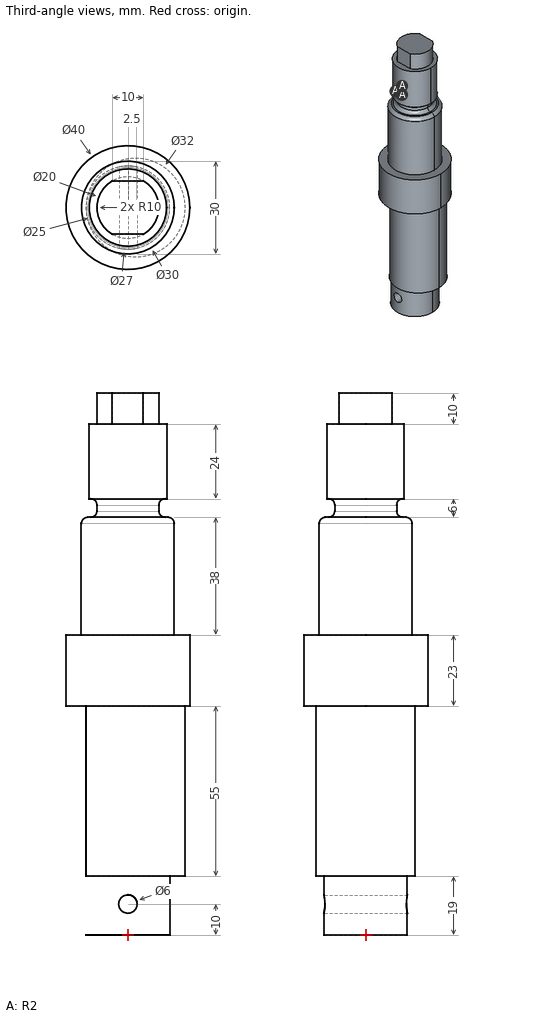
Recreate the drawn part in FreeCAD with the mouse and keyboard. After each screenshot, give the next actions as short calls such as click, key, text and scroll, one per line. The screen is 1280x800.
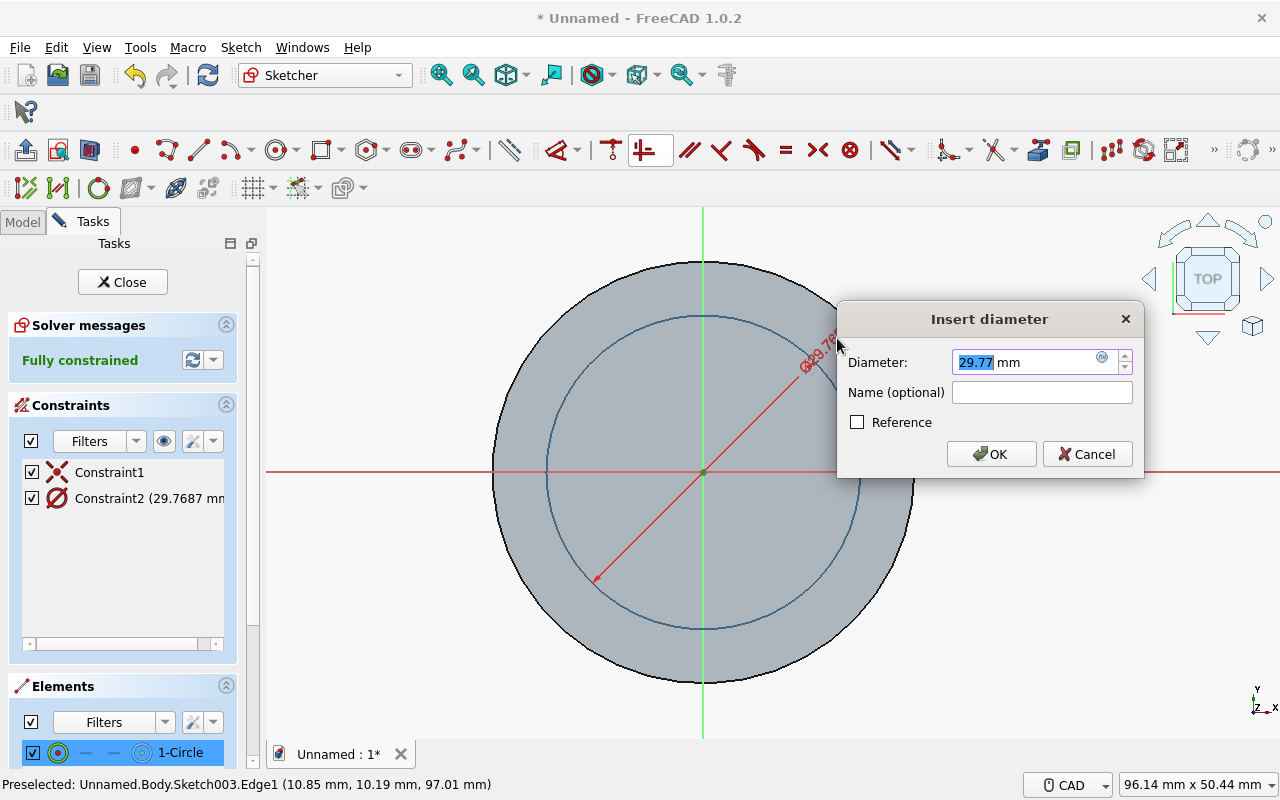
text(30)
key(Return)
key(Escape)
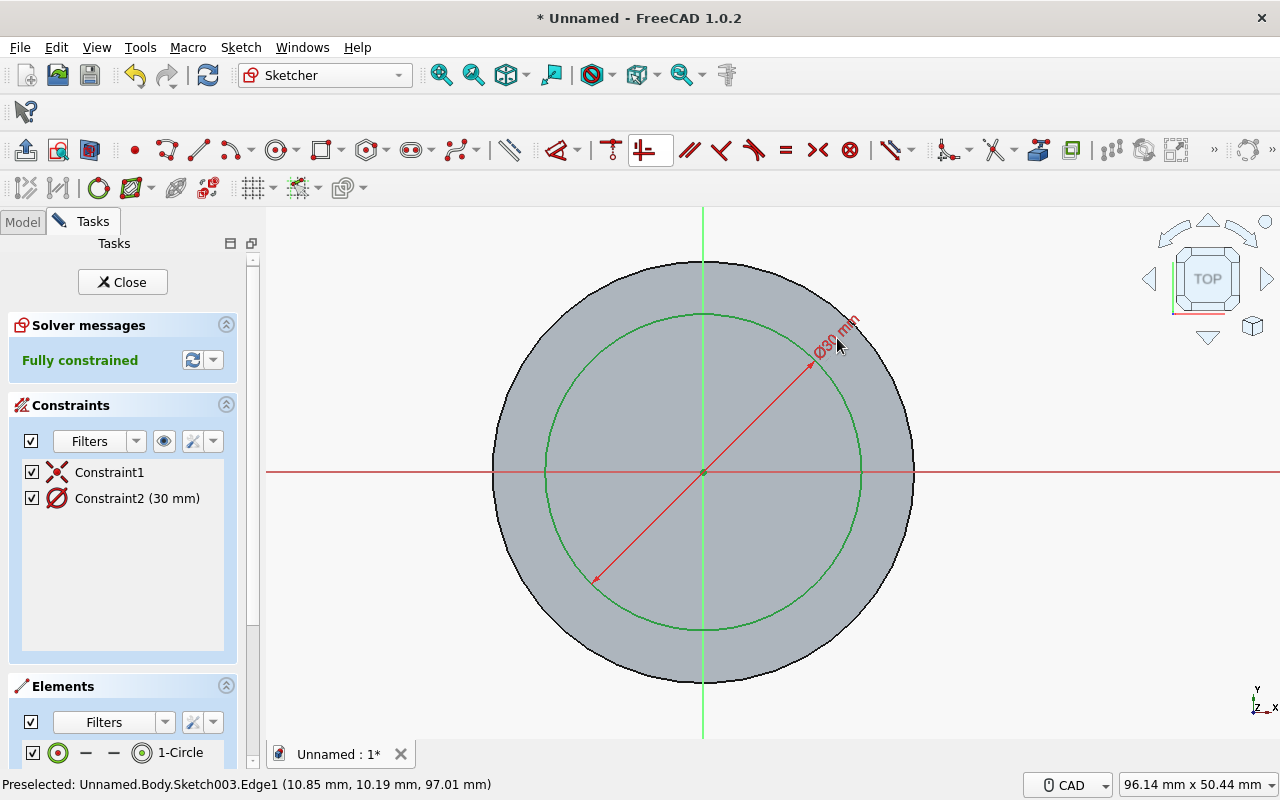
click(123, 282)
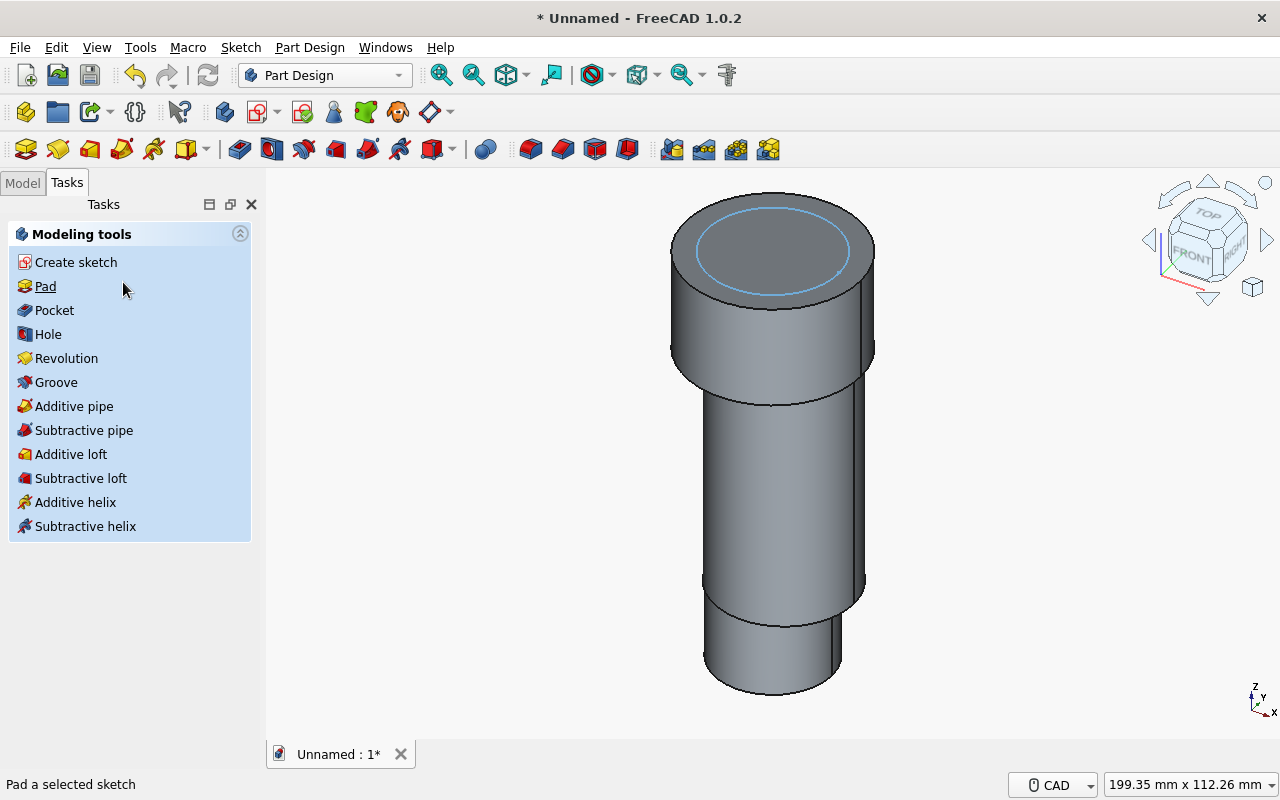
click(26, 150)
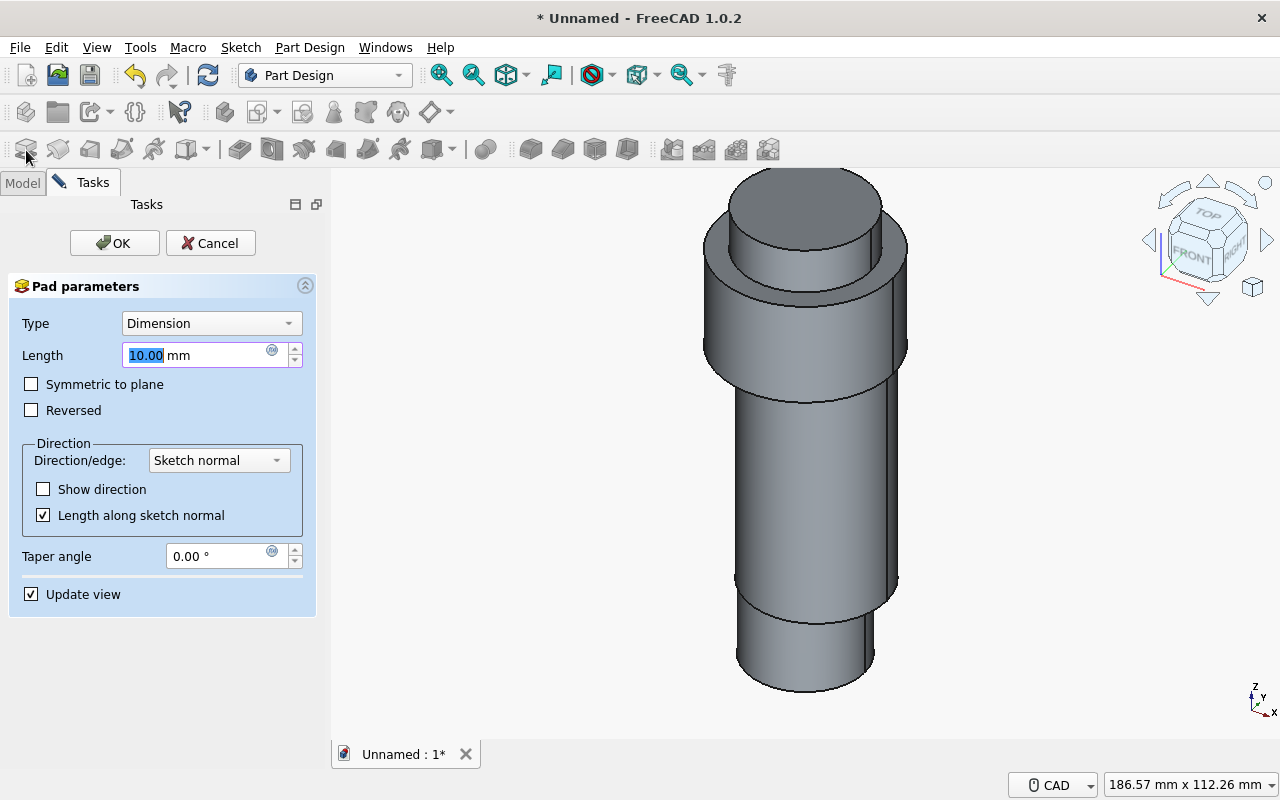
text(38)
key(Tab)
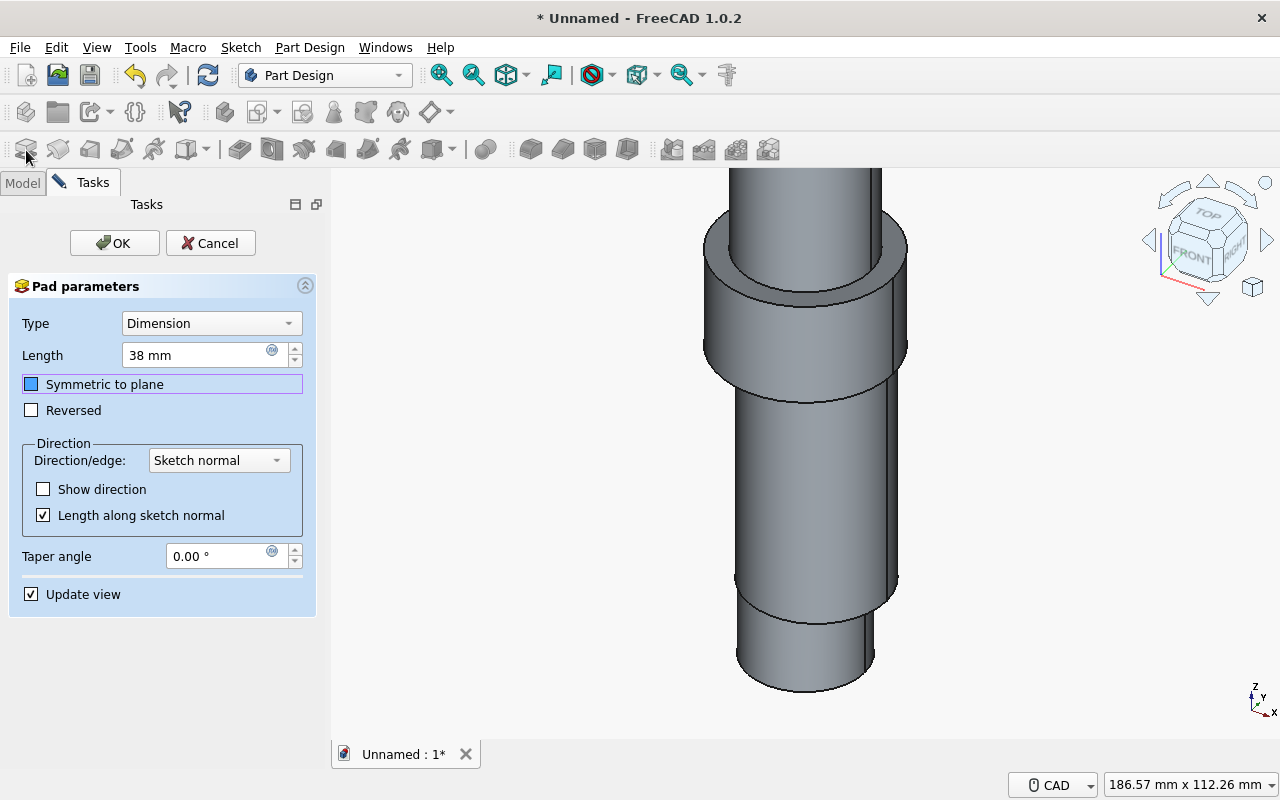
click(115, 243)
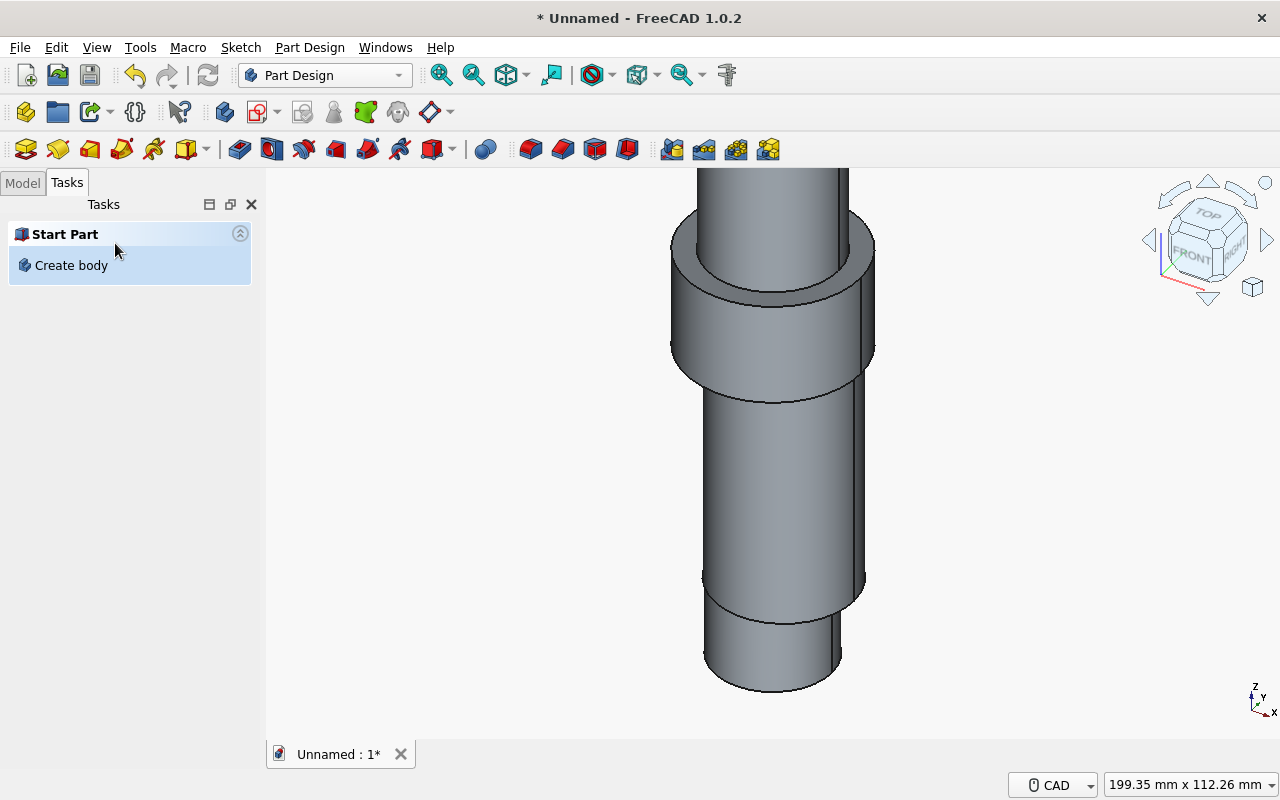
key(v)
key(f)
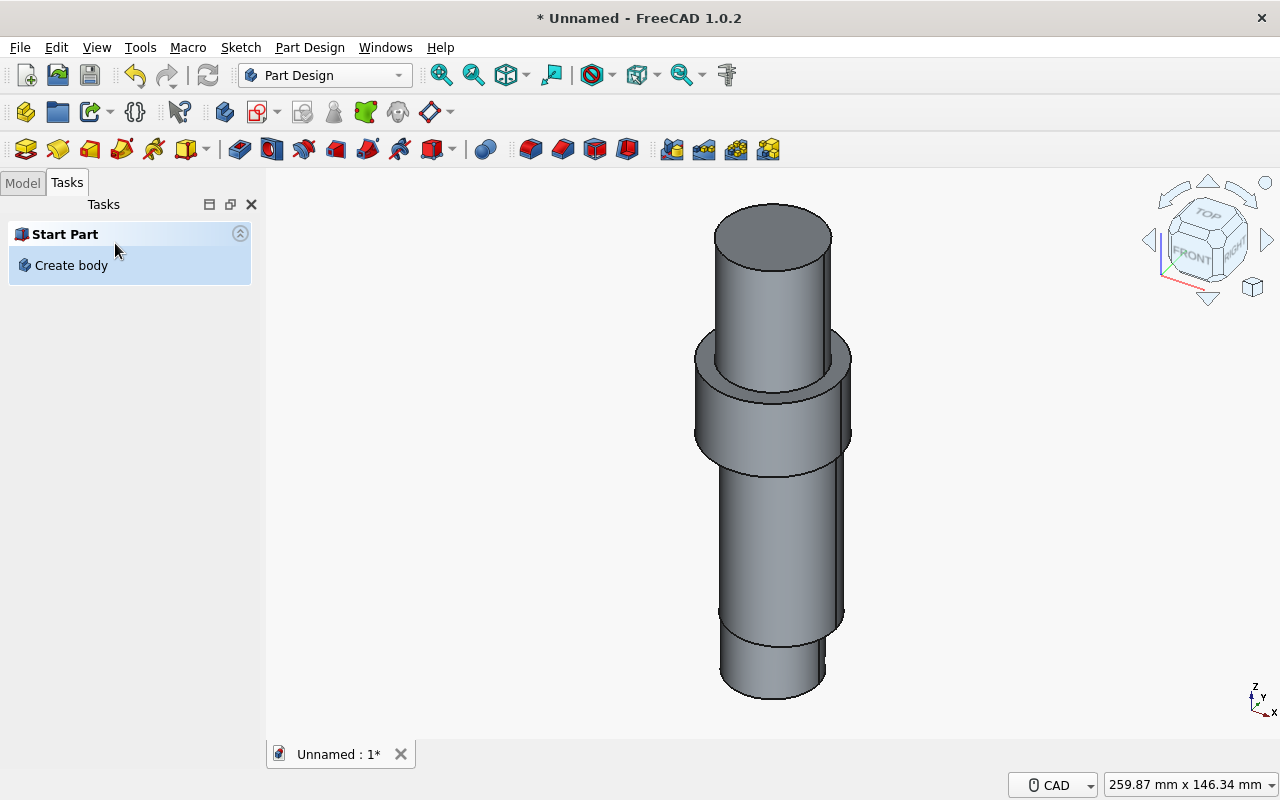
click(773, 237)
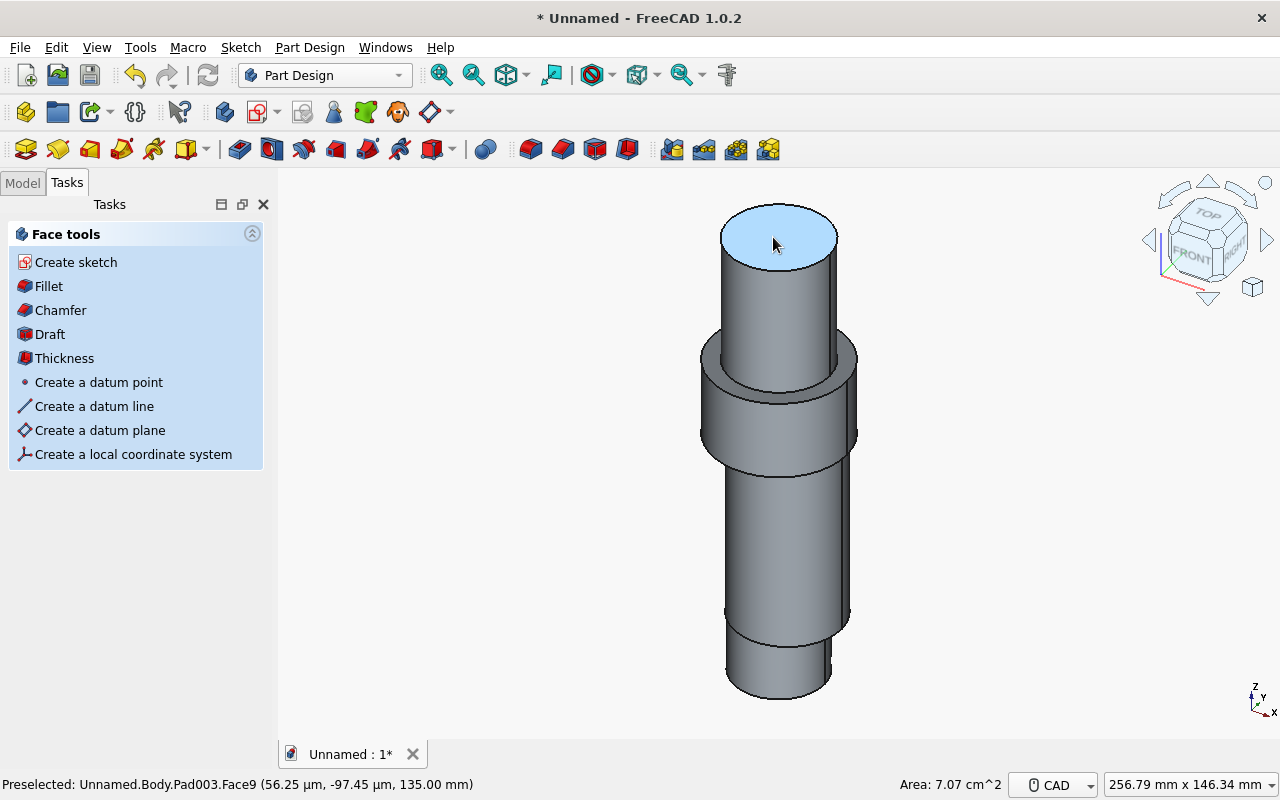
click(258, 112)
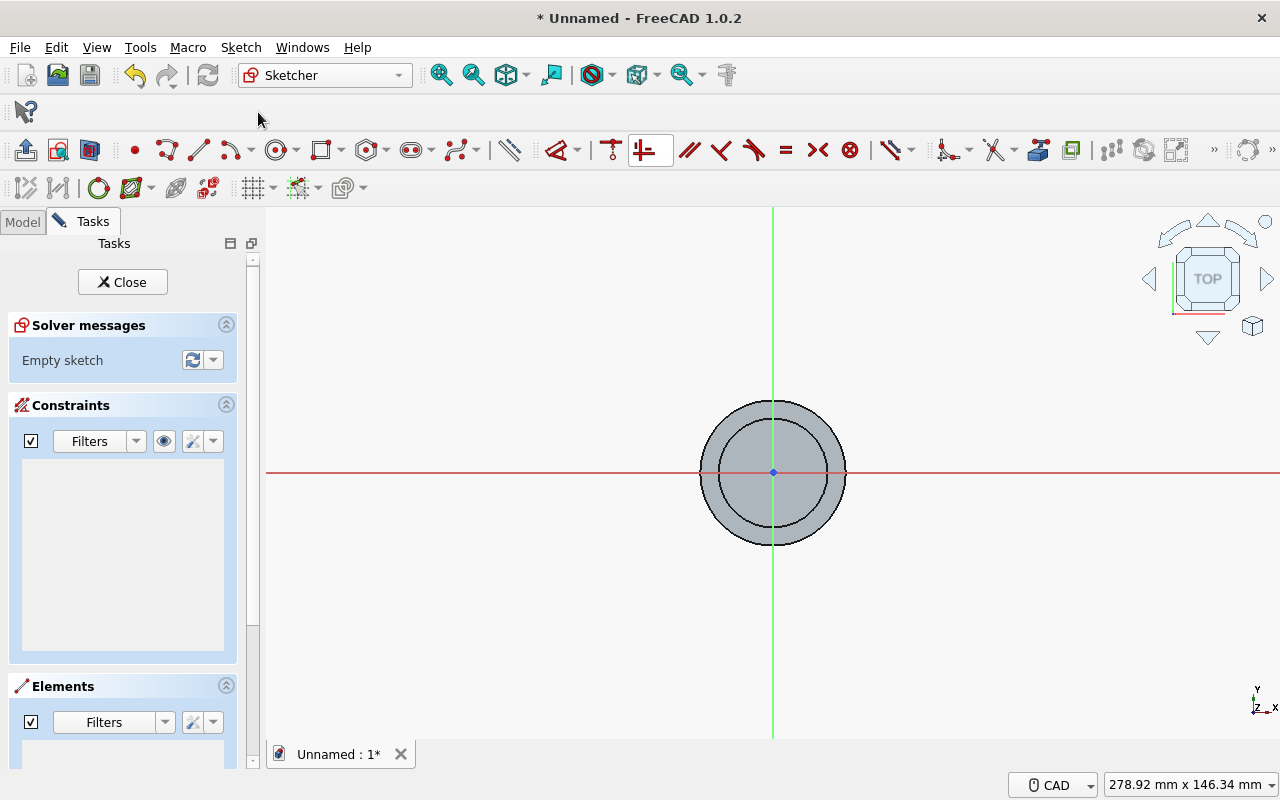
scroll(790, 473, up, 8)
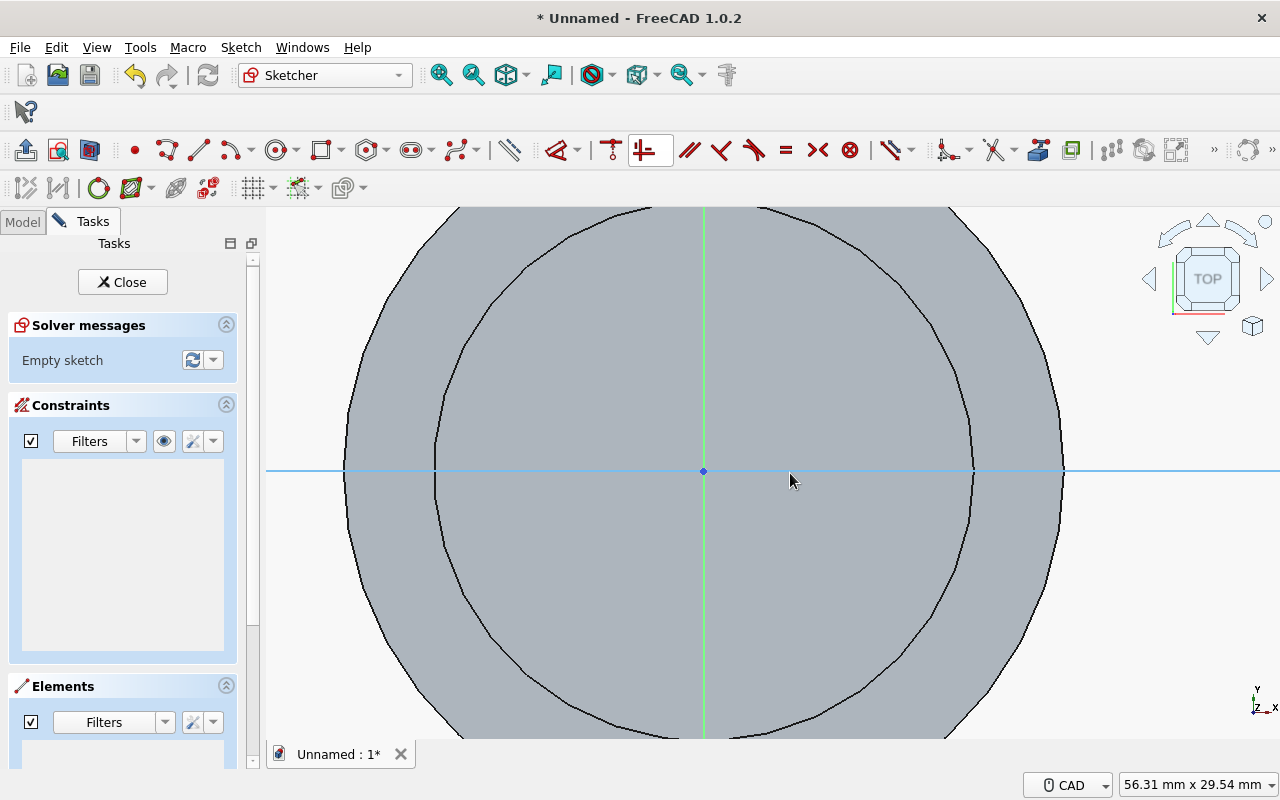
key(g)
key(c)